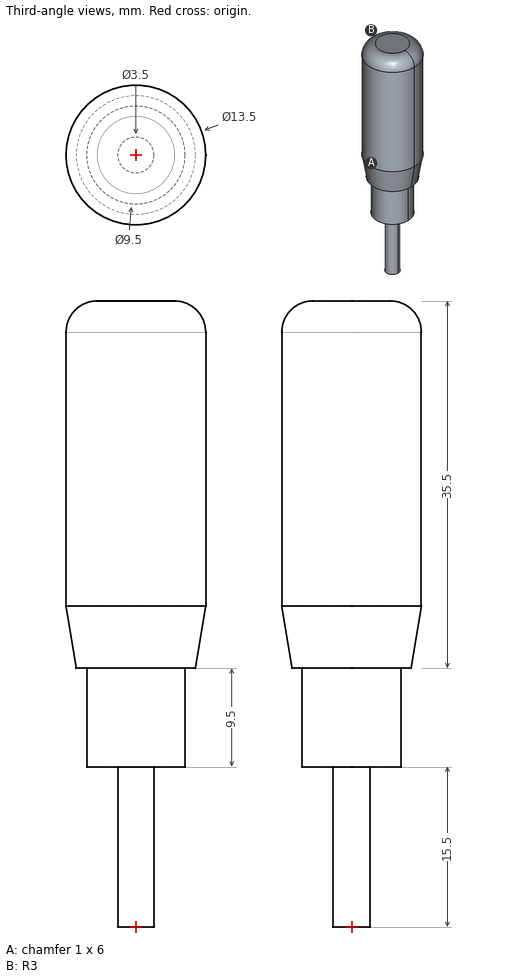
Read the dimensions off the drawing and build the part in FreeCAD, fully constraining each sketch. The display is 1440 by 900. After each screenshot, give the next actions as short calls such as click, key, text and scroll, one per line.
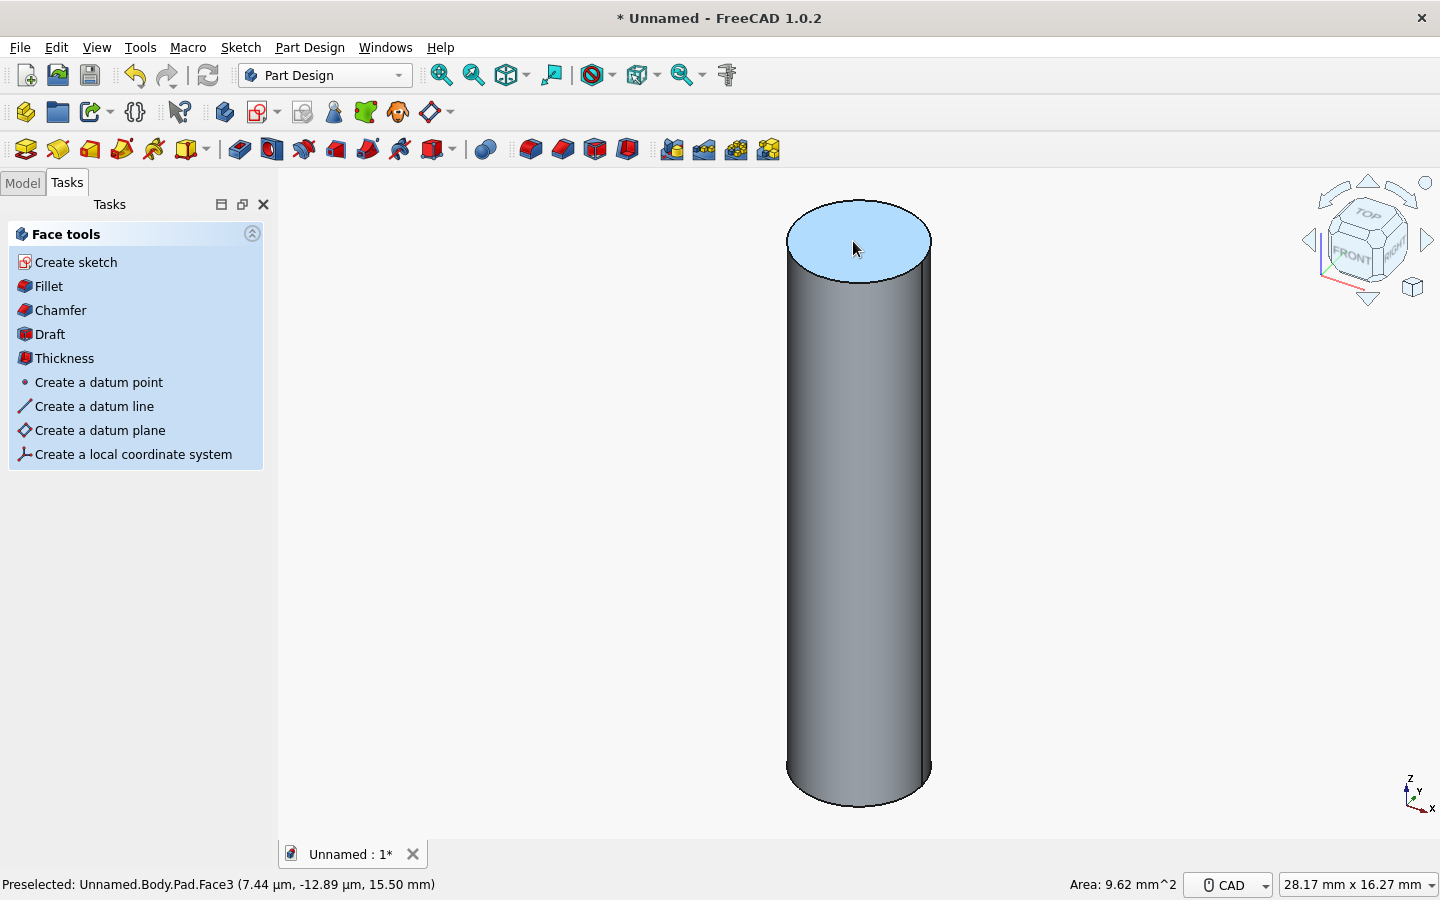
click(258, 112)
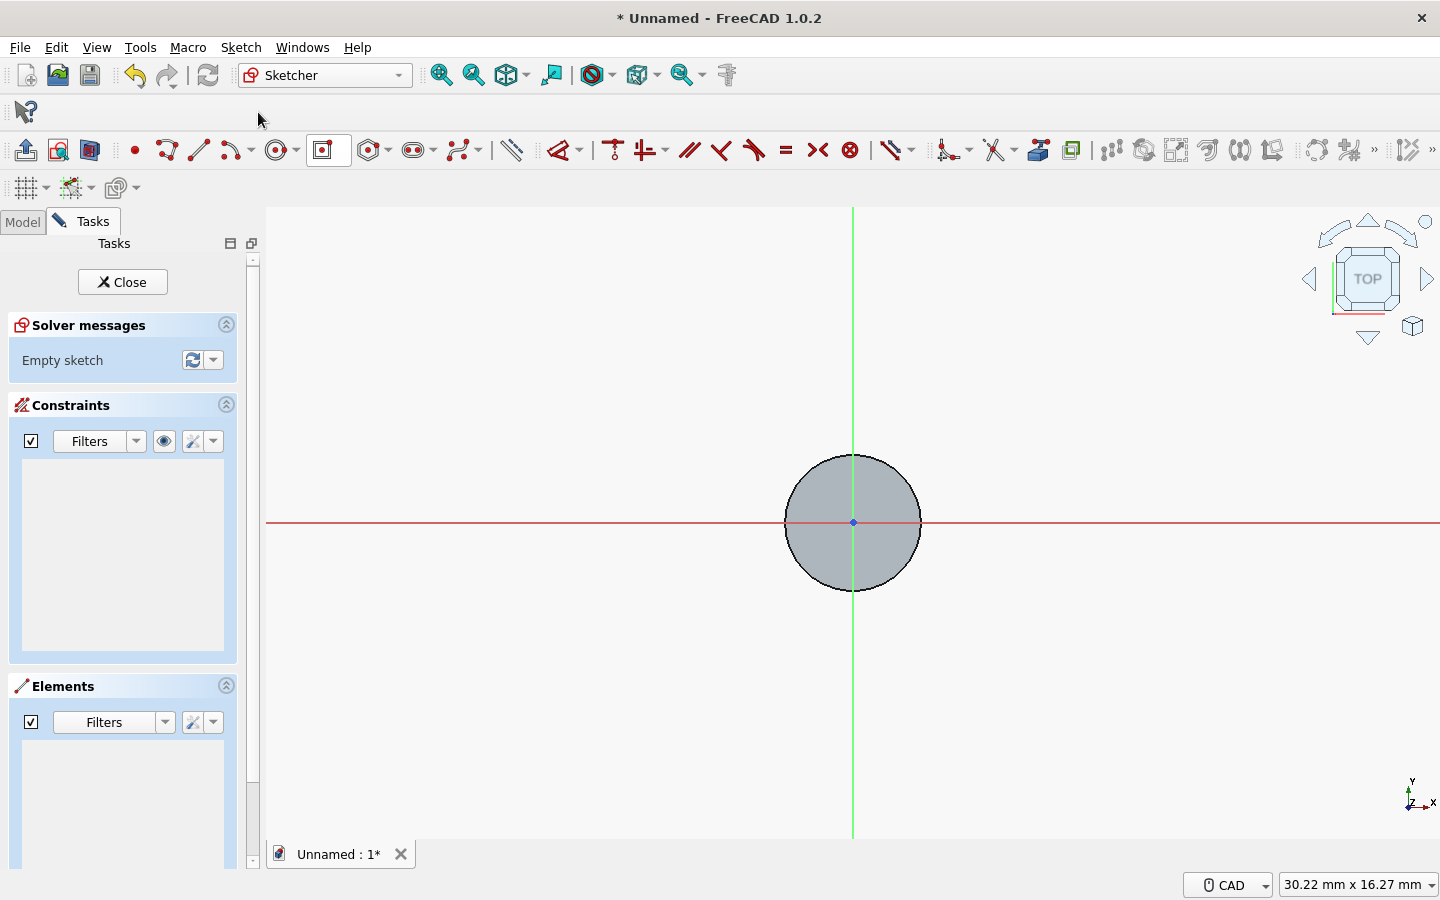
click(276, 150)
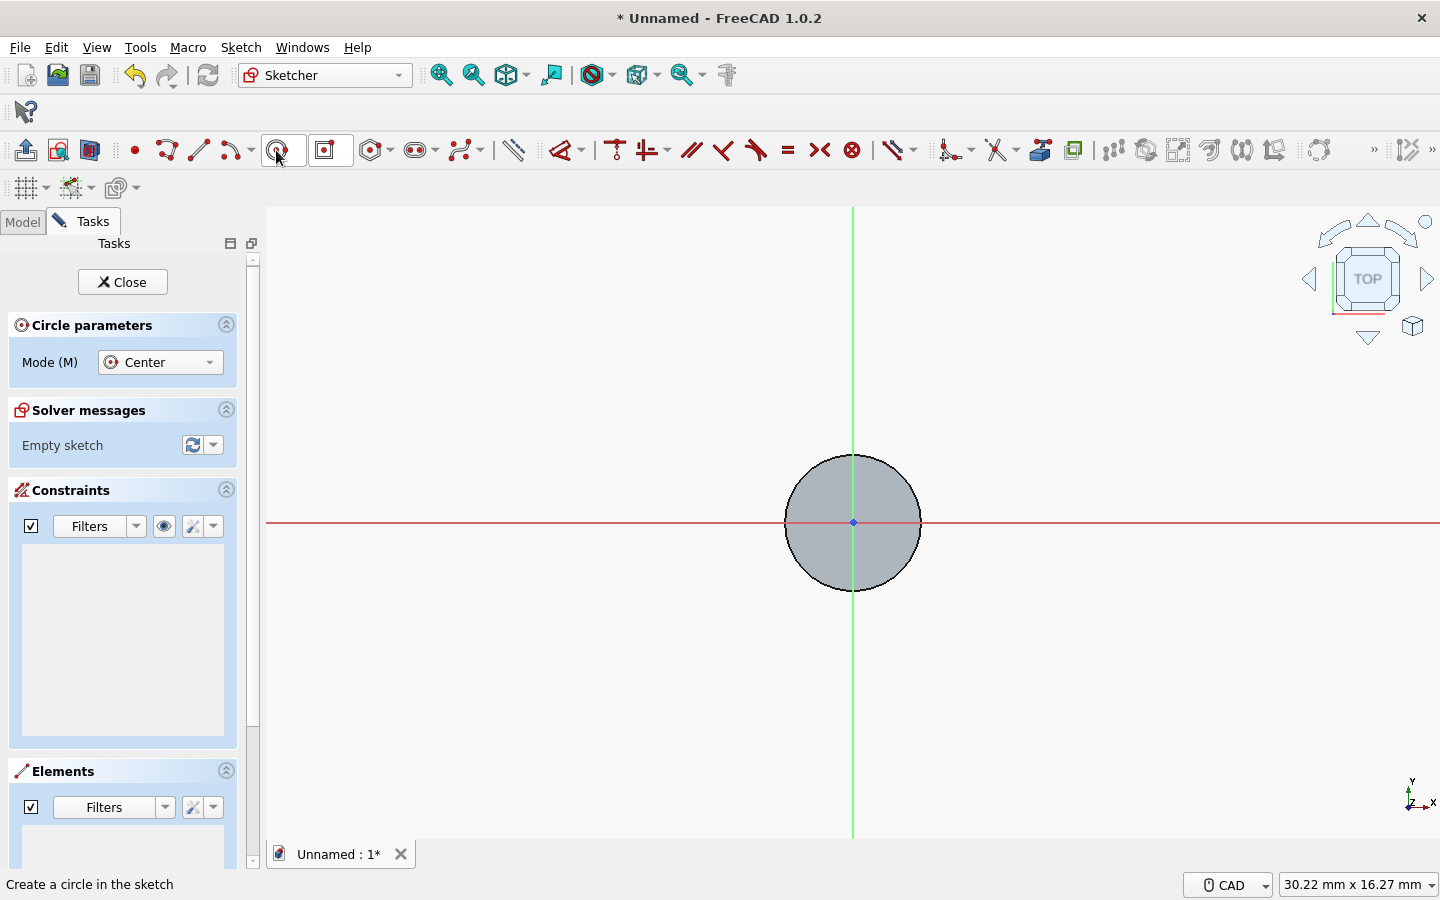
click(853, 523)
click(983, 393)
key(Escape)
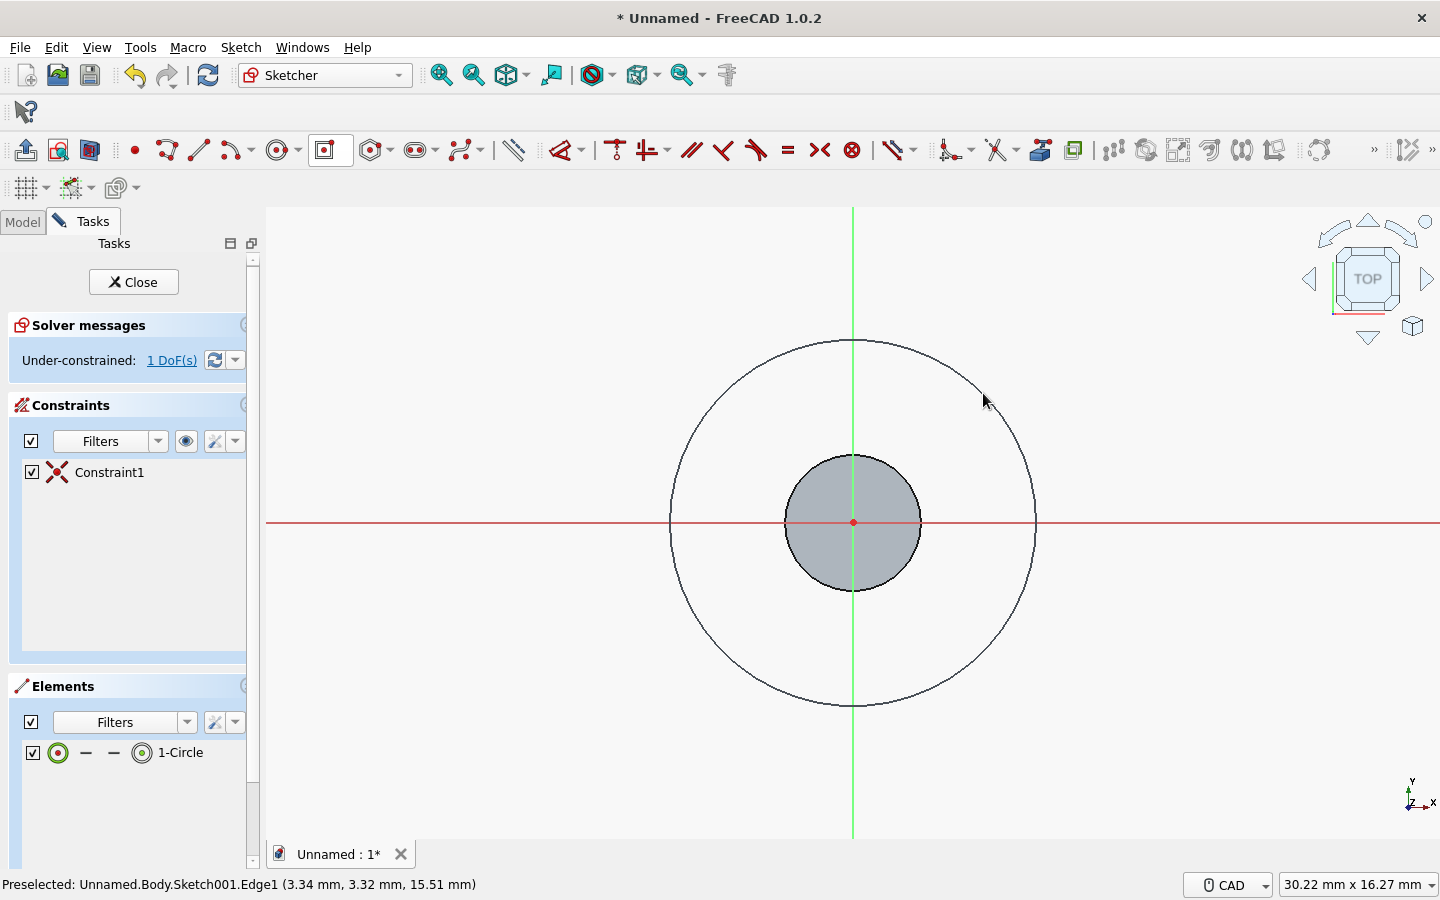
click(560, 150)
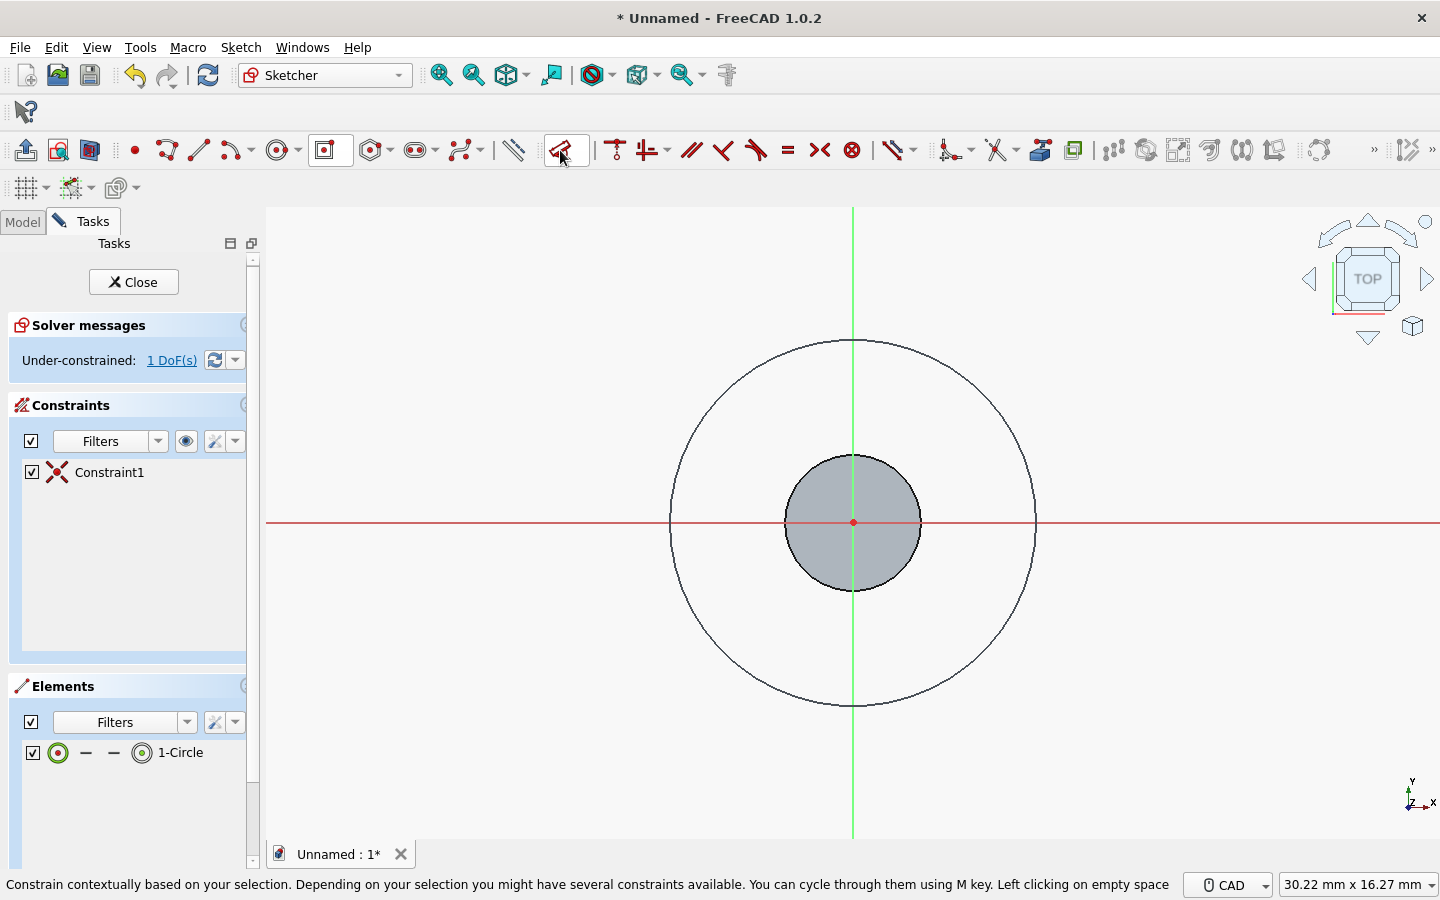
click(982, 393)
click(1005, 370)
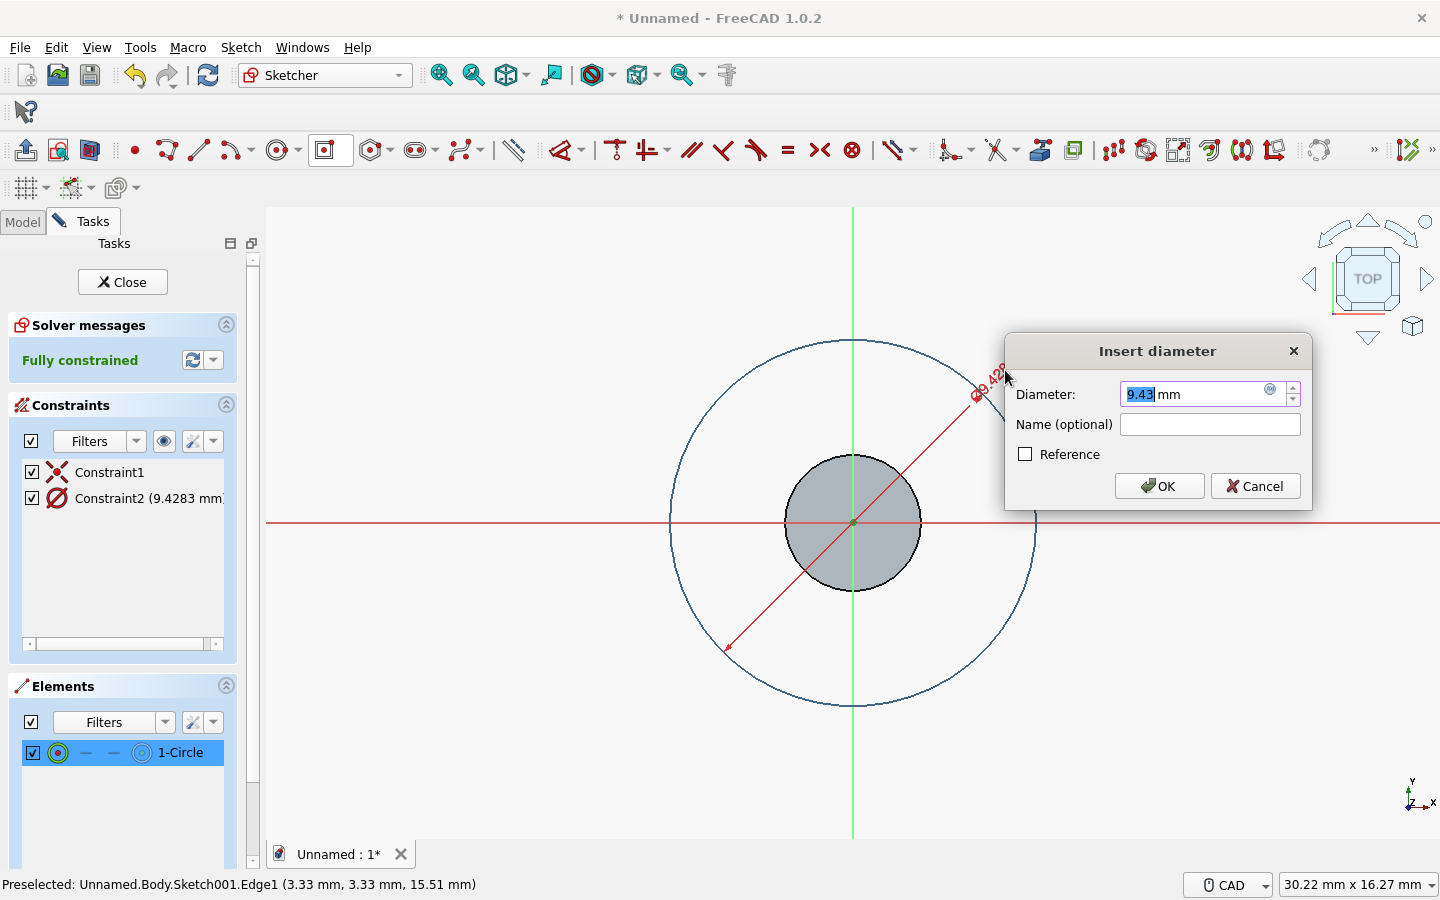
text(9.5)
key(Return)
key(Escape)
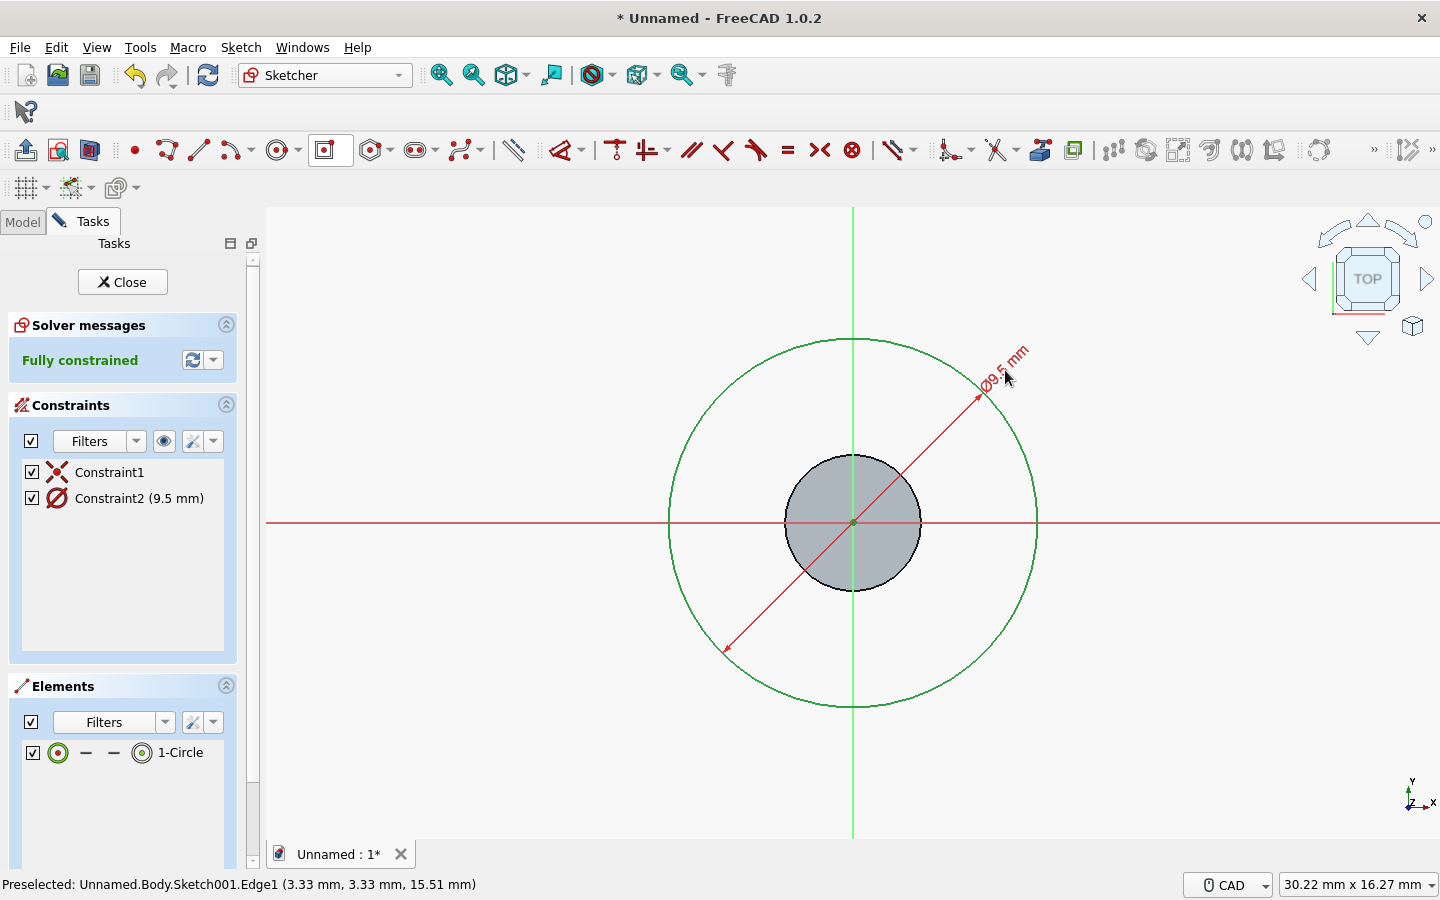
click(123, 282)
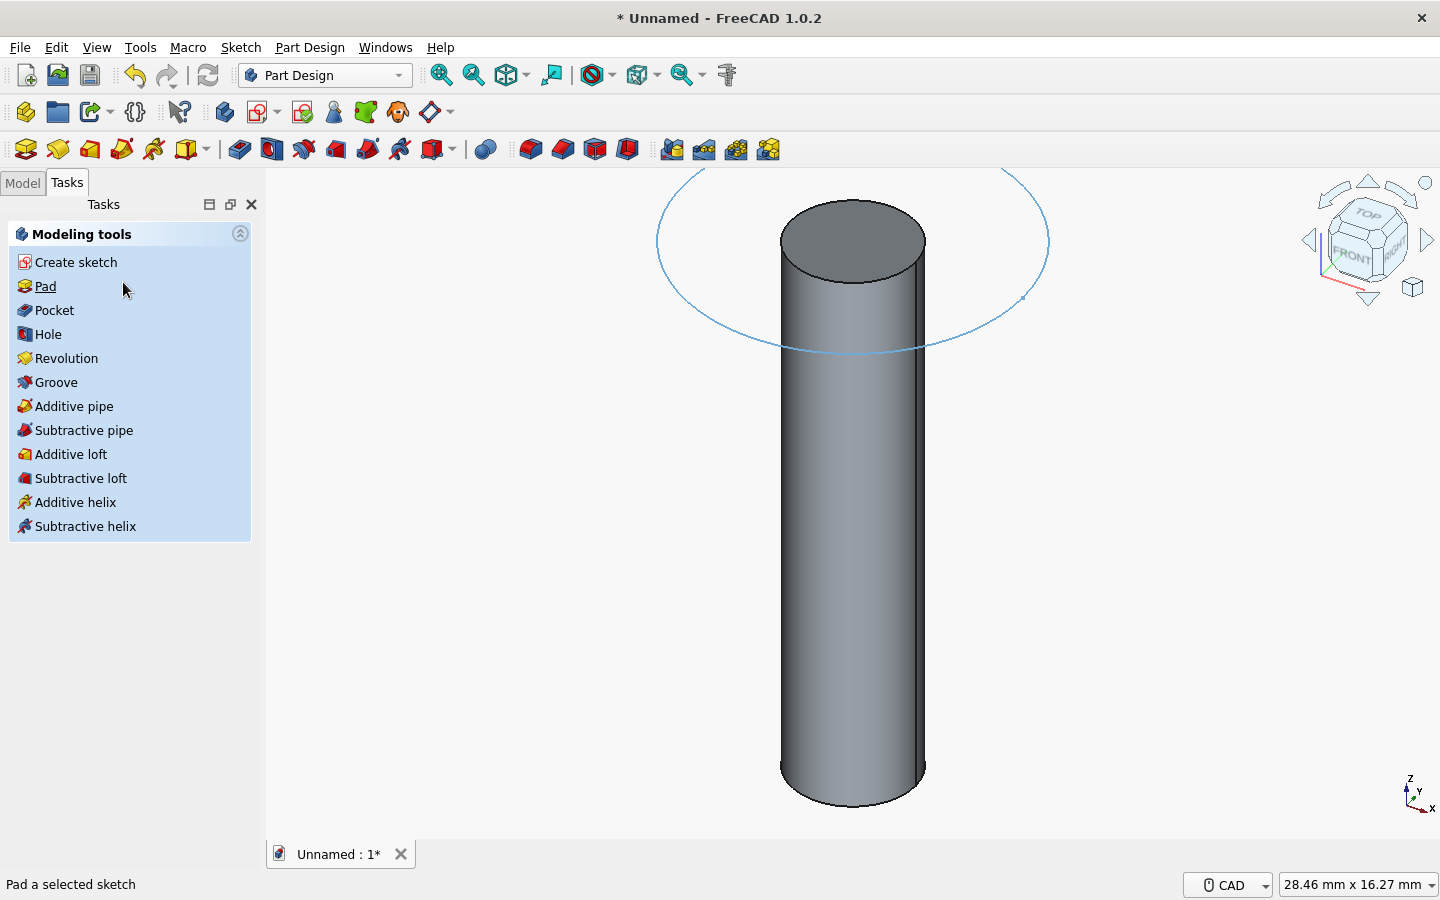
click(26, 150)